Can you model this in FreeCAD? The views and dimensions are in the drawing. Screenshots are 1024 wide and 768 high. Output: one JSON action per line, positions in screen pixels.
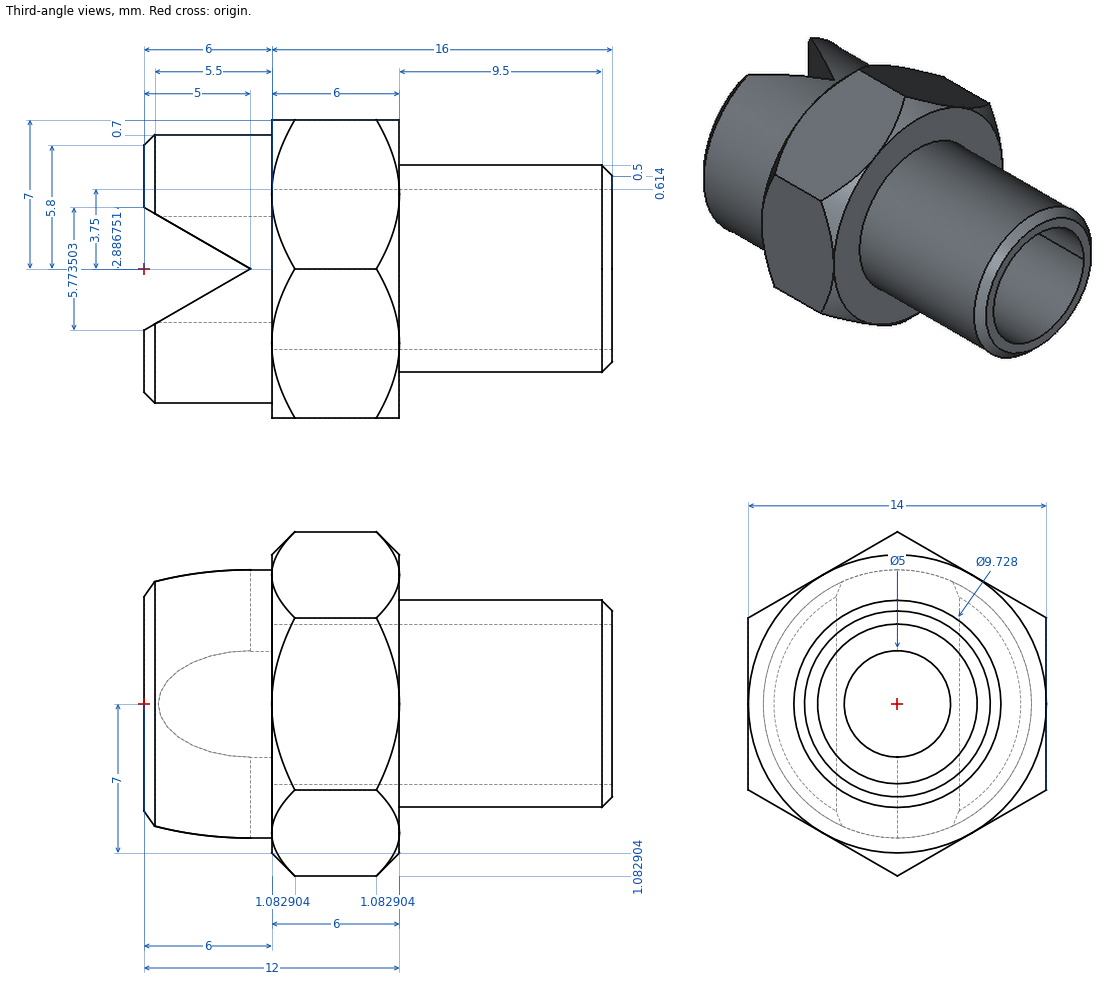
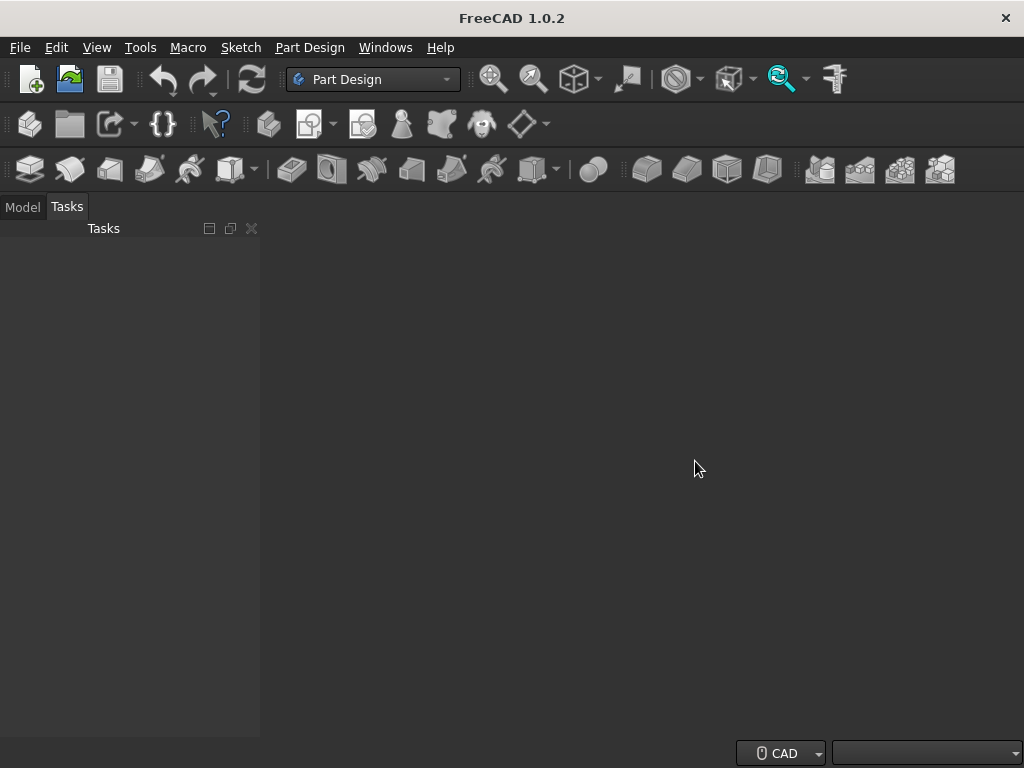
{"action": "left_click", "coordinate": [30, 80]}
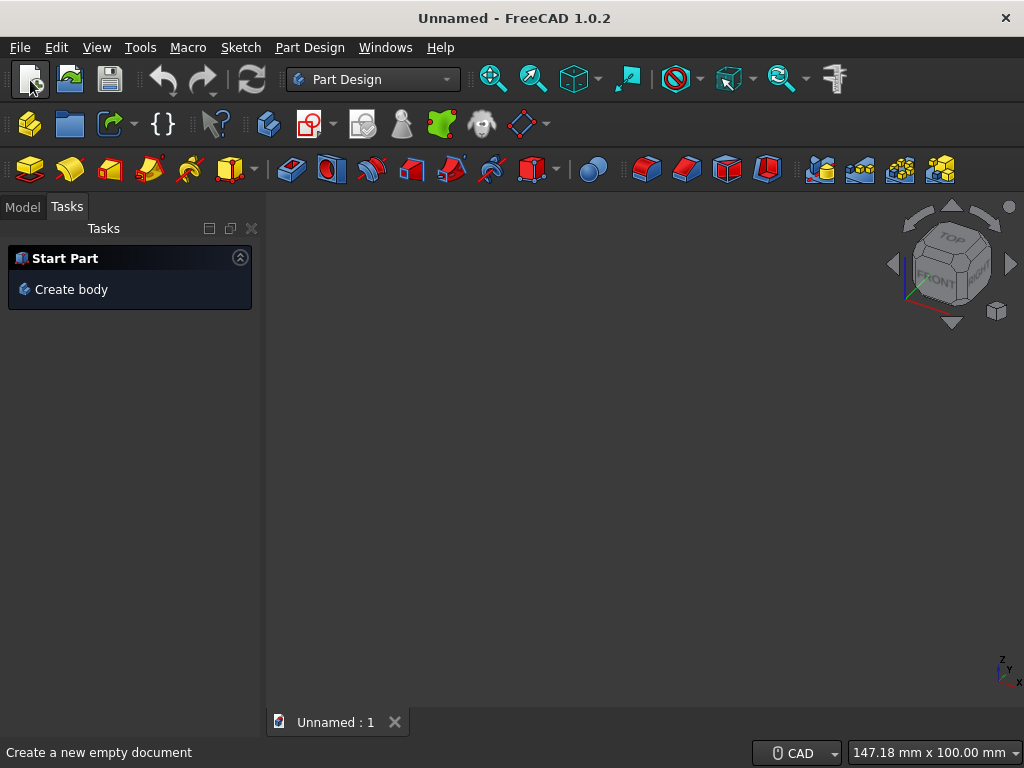
{"action": "left_click", "coordinate": [310, 124]}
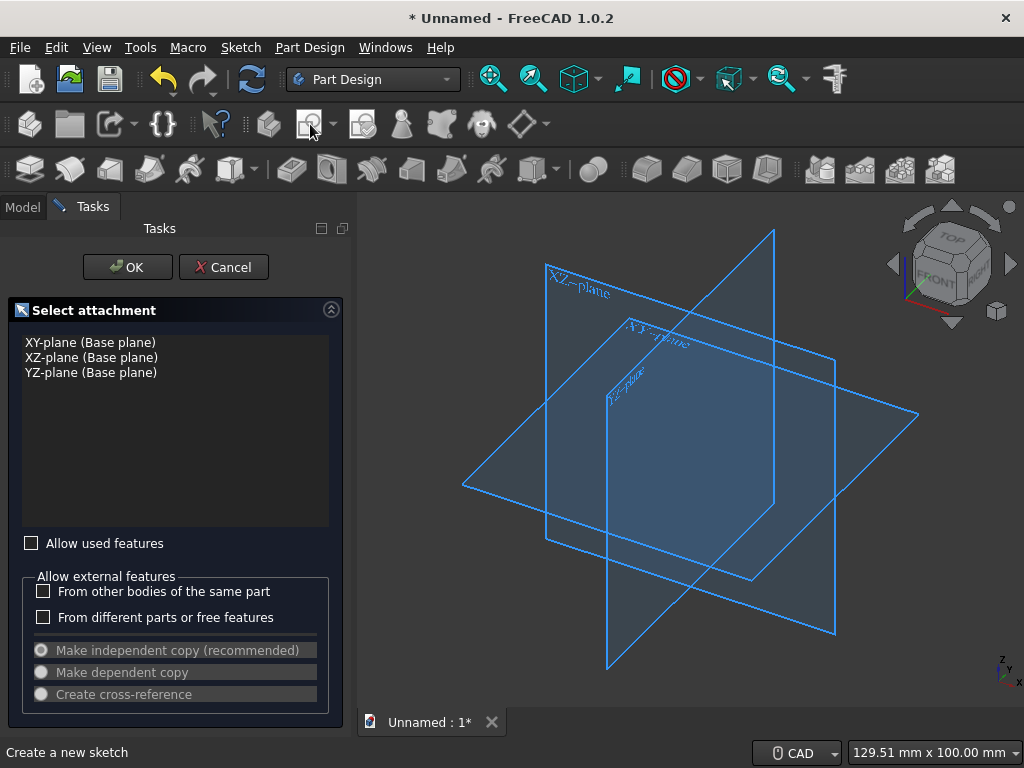
{"action": "left_click", "coordinate": [82, 342]}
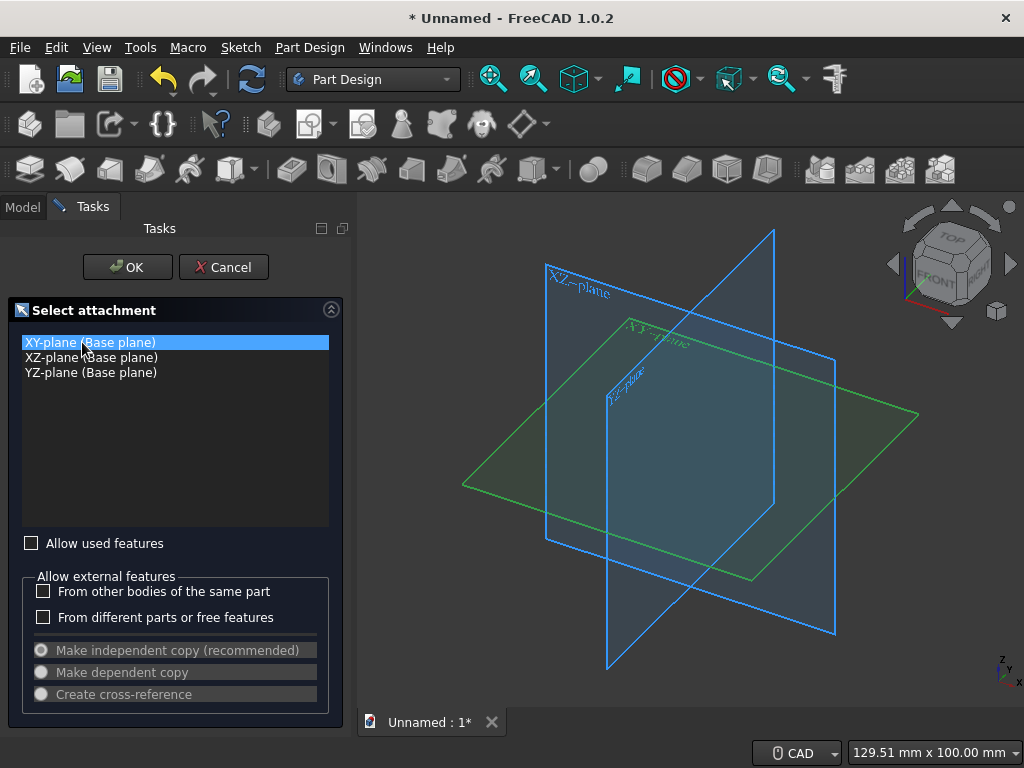
{"action": "left_click", "coordinate": [128, 267]}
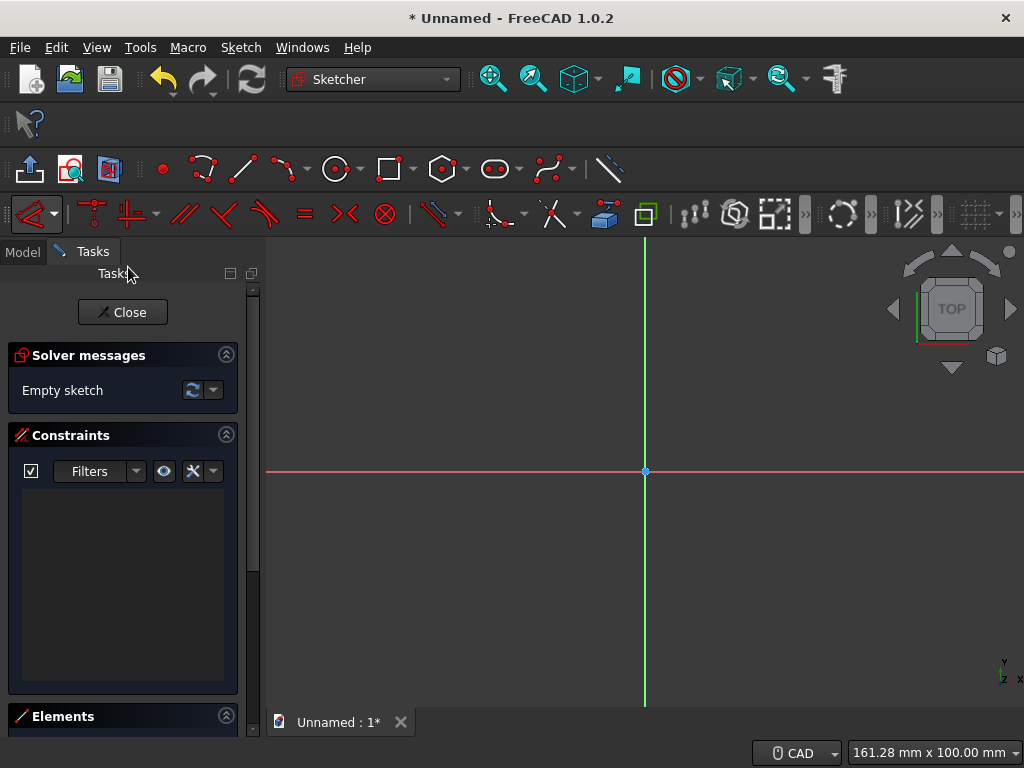
{"action": "scroll", "coordinate": [736, 450], "scroll_direction": "up", "scroll_amount": 7}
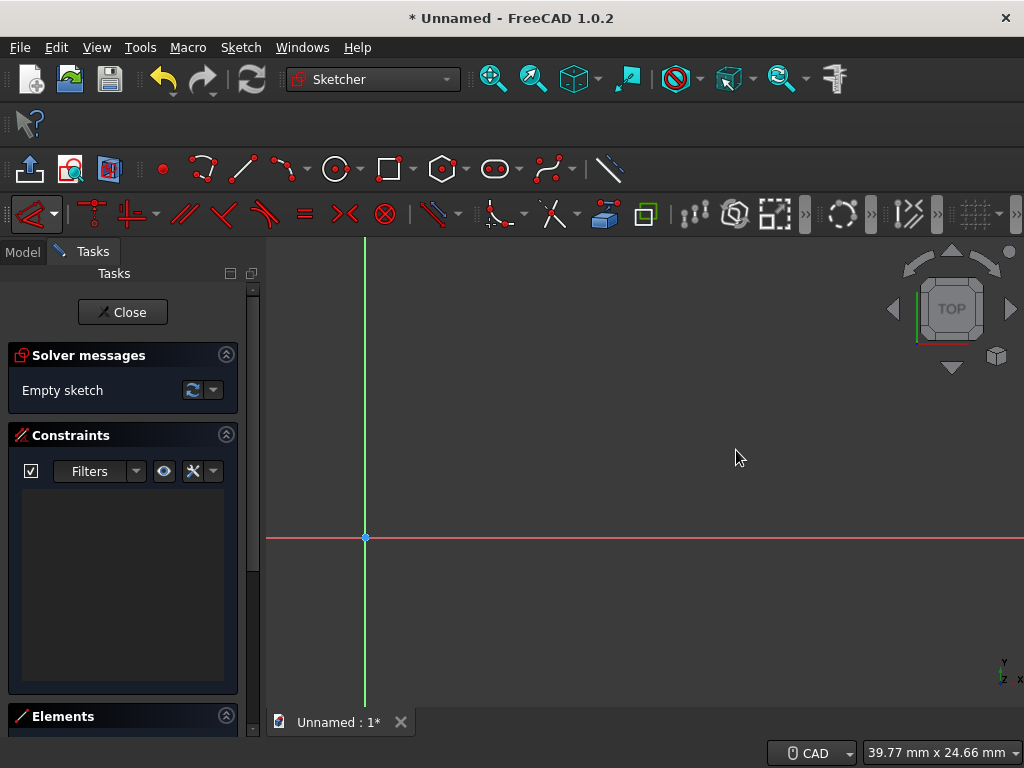
{"action": "left_click", "coordinate": [204, 170]}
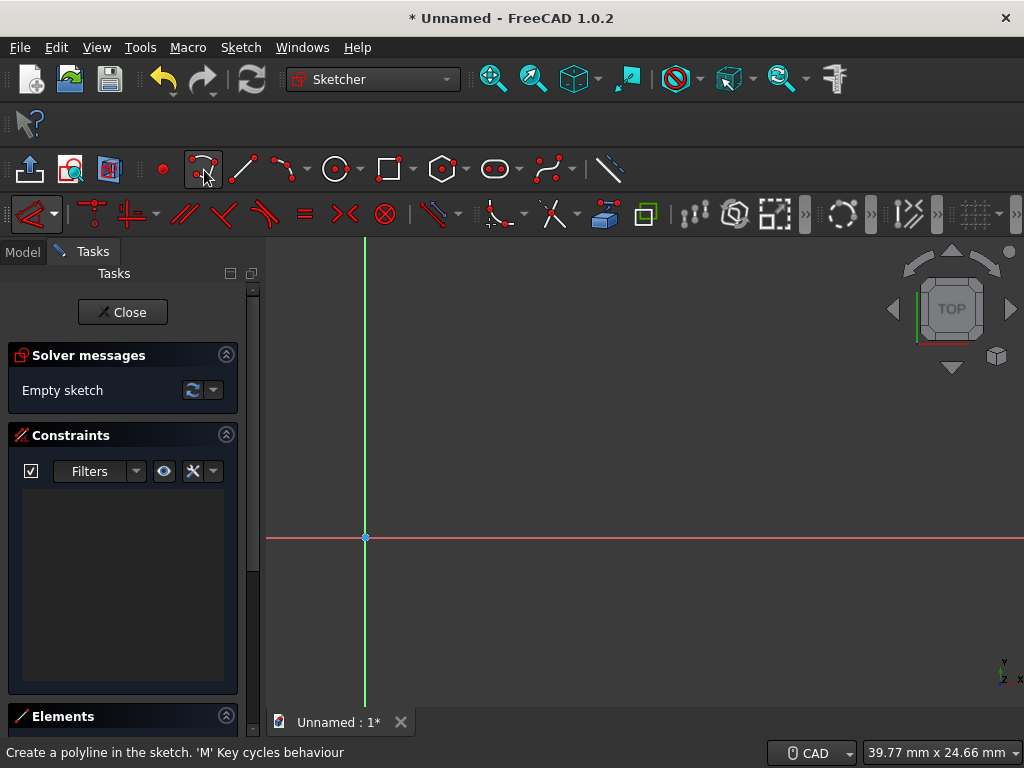
{"action": "left_click", "coordinate": [365, 538]}
{"action": "left_click", "coordinate": [479, 529]}
{"action": "left_click", "coordinate": [479, 466]}
{"action": "left_click", "coordinate": [784, 466]}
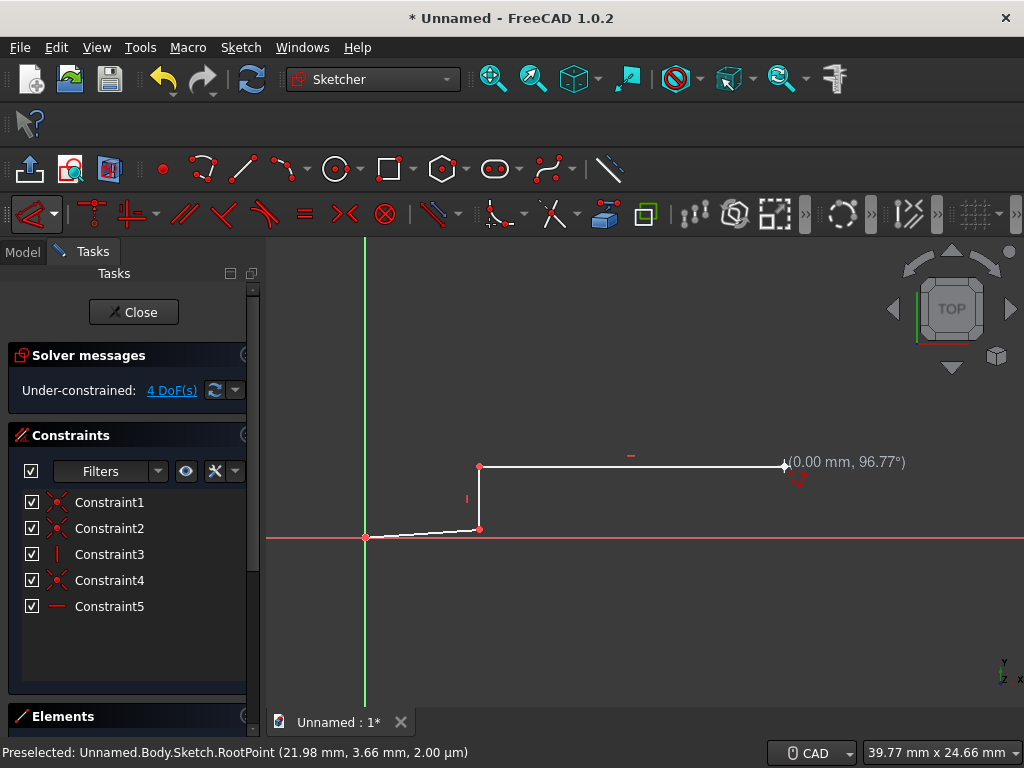
{"action": "scroll", "coordinate": [784, 455], "scroll_direction": "up", "scroll_amount": 2}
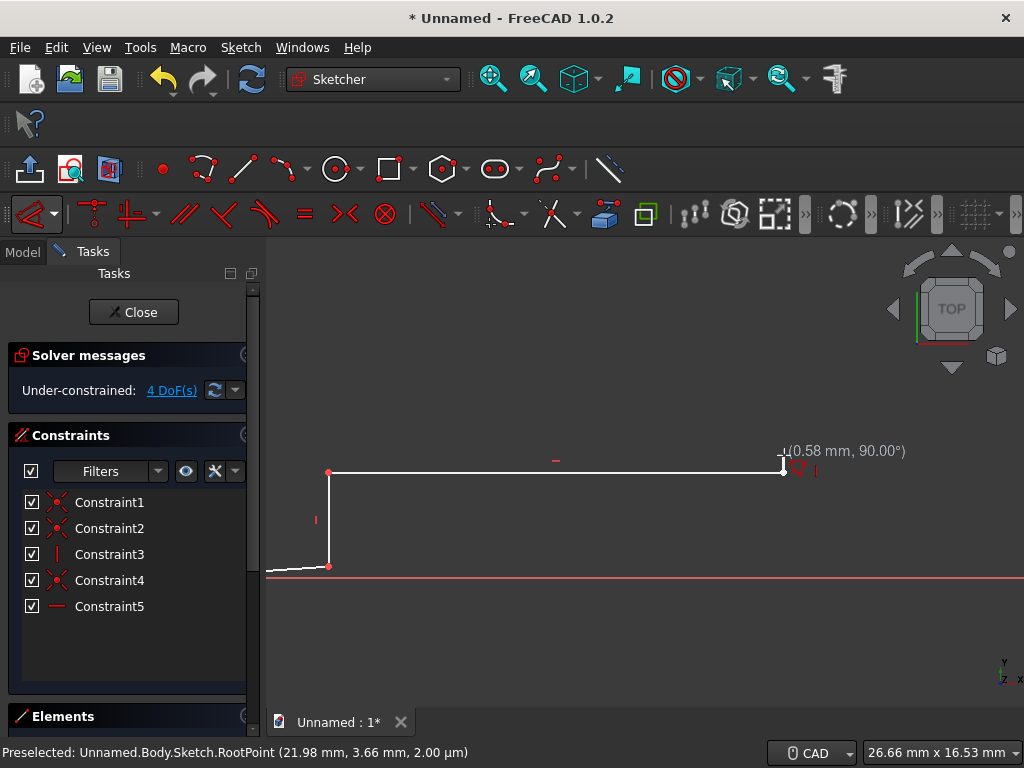
{"action": "left_click", "coordinate": [784, 454]}
{"action": "left_click", "coordinate": [770, 440]}
{"action": "left_click", "coordinate": [500, 440]}
{"action": "left_click", "coordinate": [500, 379]}
{"action": "left_click", "coordinate": [329, 379]}
{"action": "left_click", "coordinate": [329, 399]}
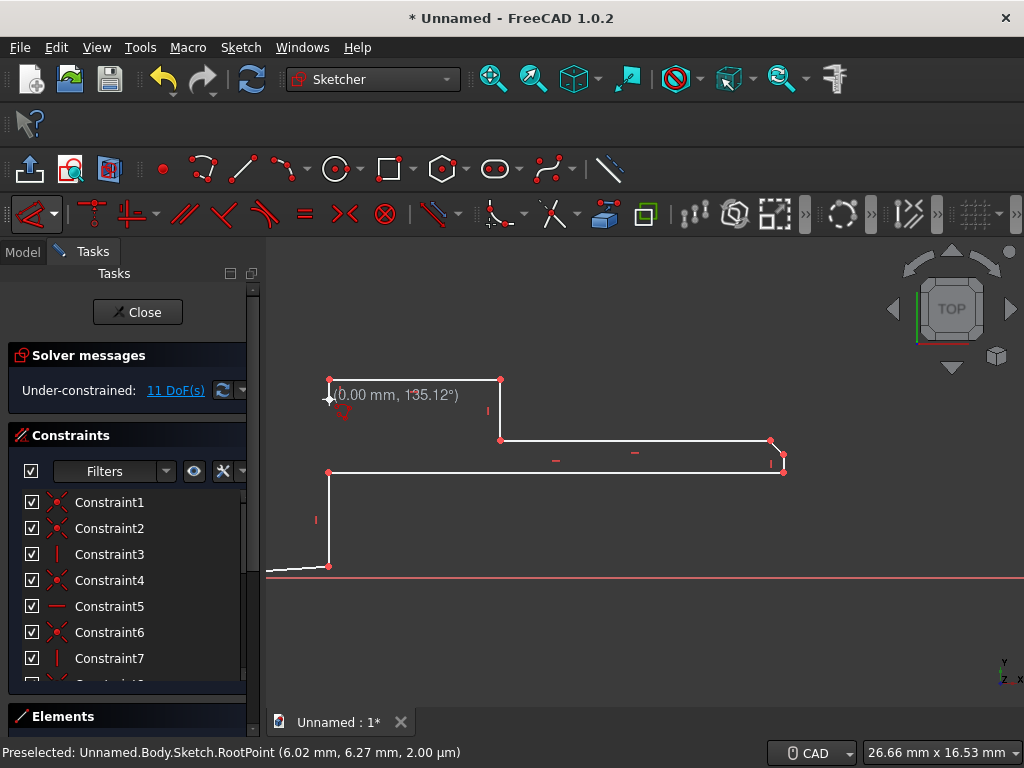
{"action": "scroll", "coordinate": [790, 458], "scroll_direction": "down", "scroll_amount": 2}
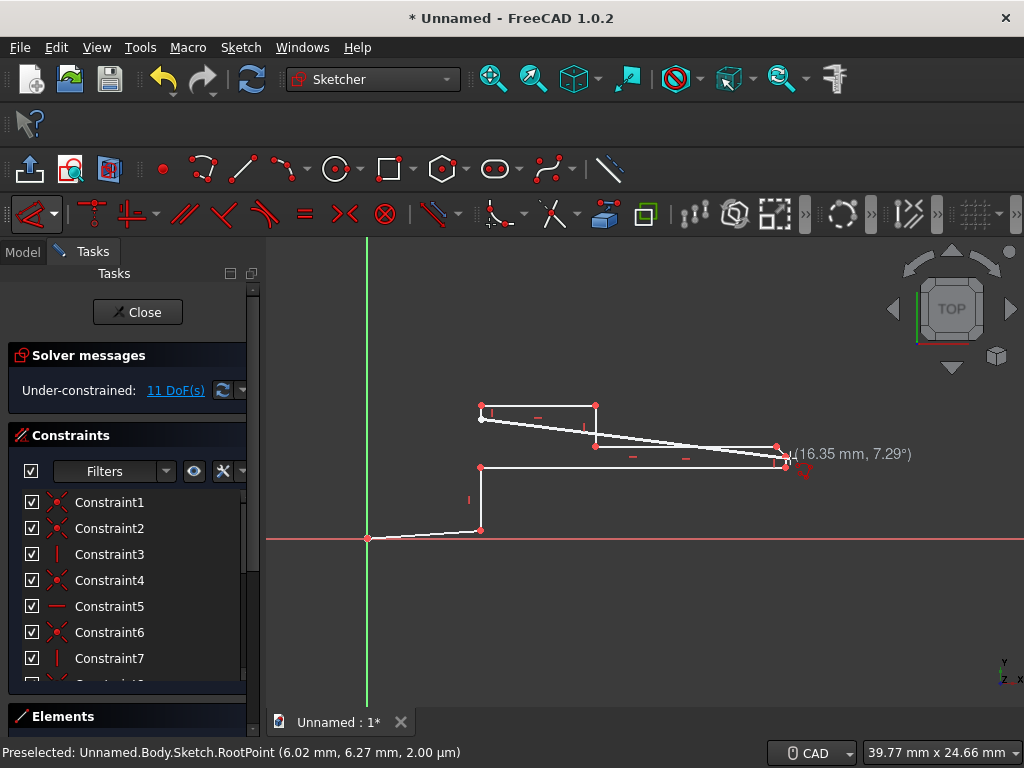
{"action": "scroll", "coordinate": [377, 419], "scroll_direction": "up", "scroll_amount": 3}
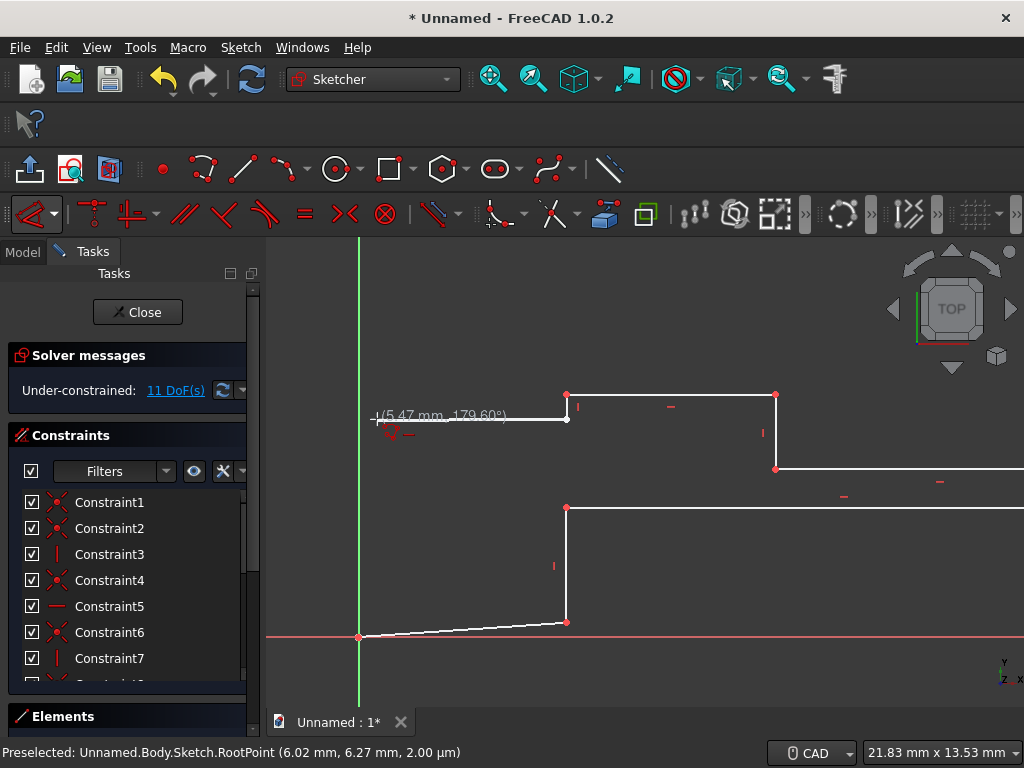
{"action": "left_click", "coordinate": [376, 418]}
{"action": "left_click", "coordinate": [368, 436]}
{"action": "left_click", "coordinate": [359, 637]}
{"action": "key", "text": "Escape"}
{"action": "key", "text": "Escape"}